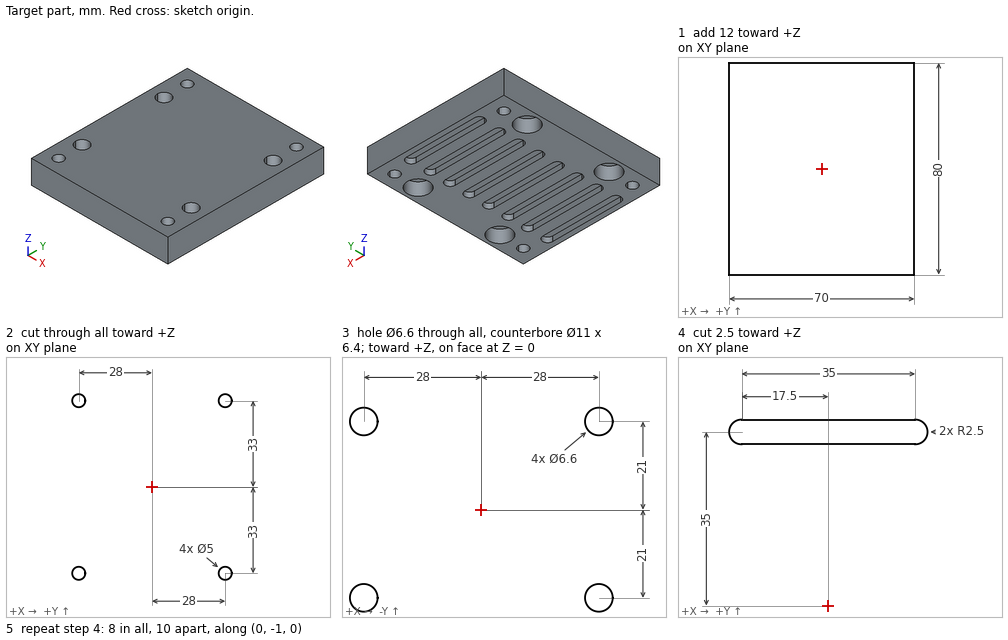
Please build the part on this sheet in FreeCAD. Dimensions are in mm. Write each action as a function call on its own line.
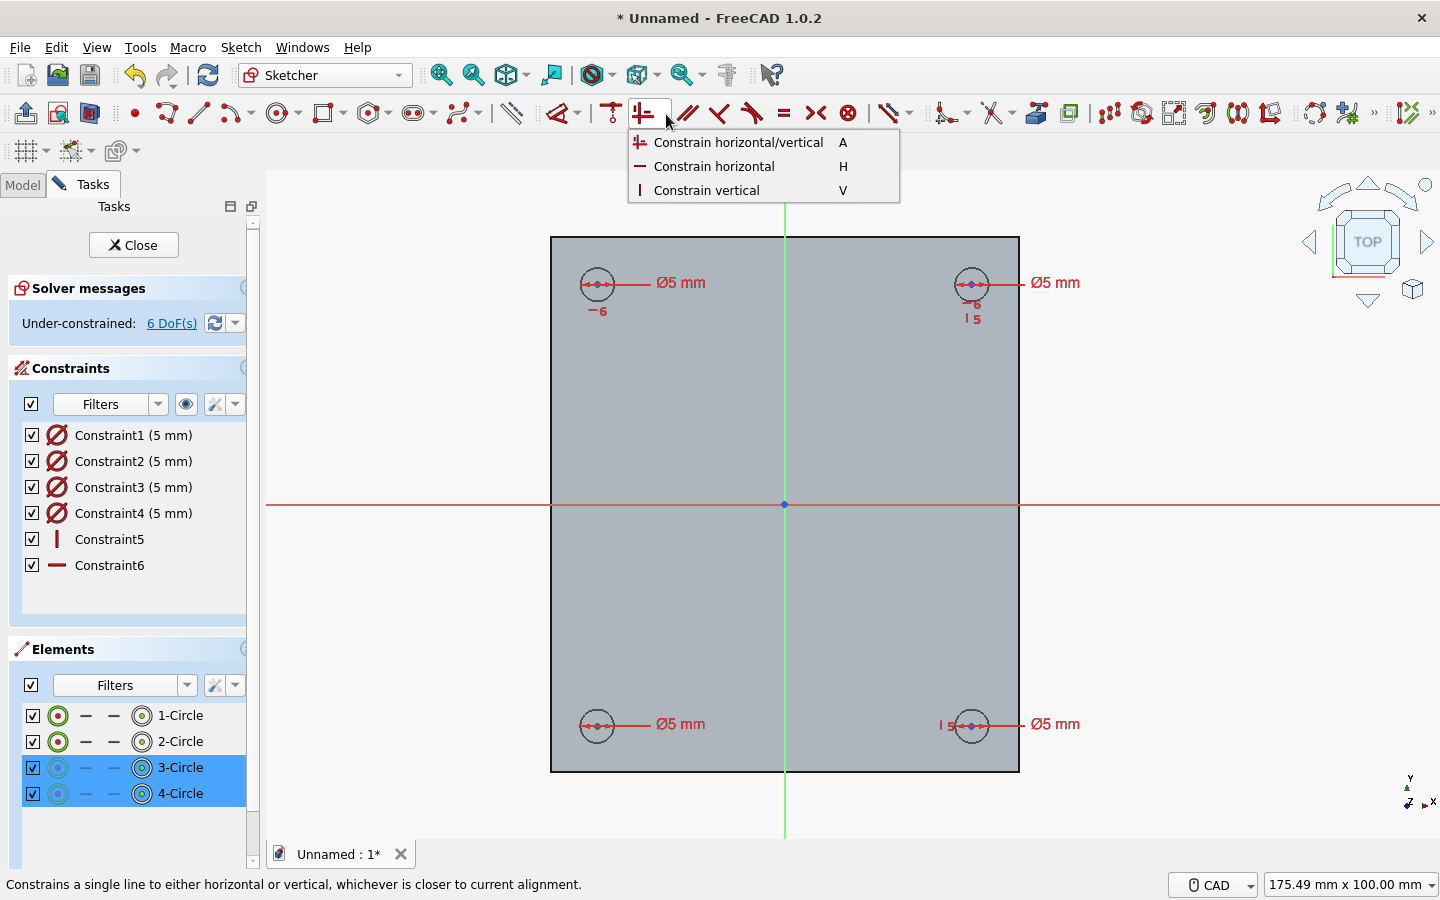
click(764, 190)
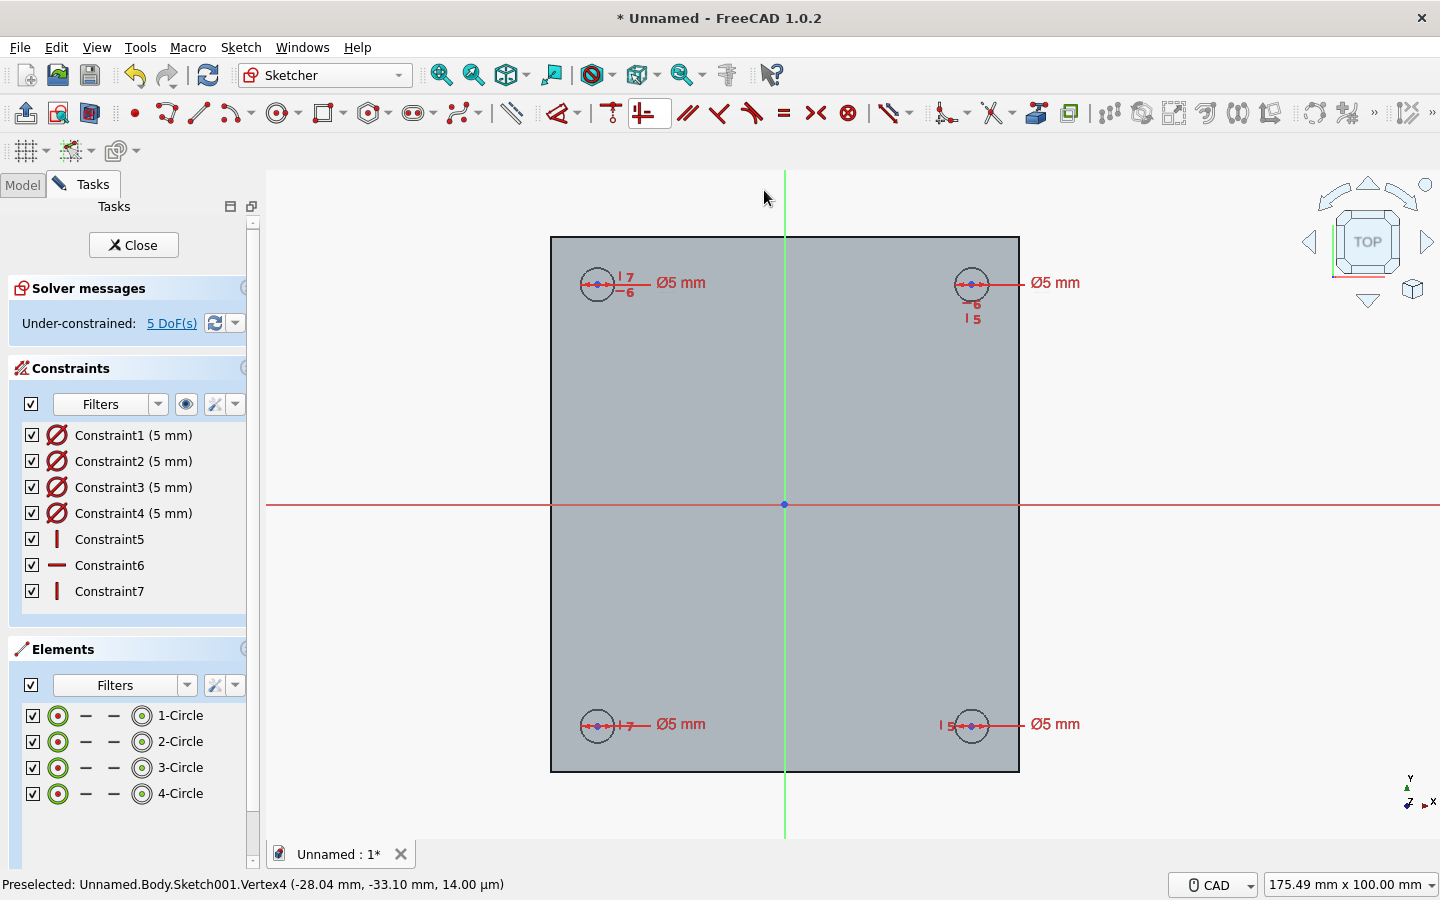
click(972, 726)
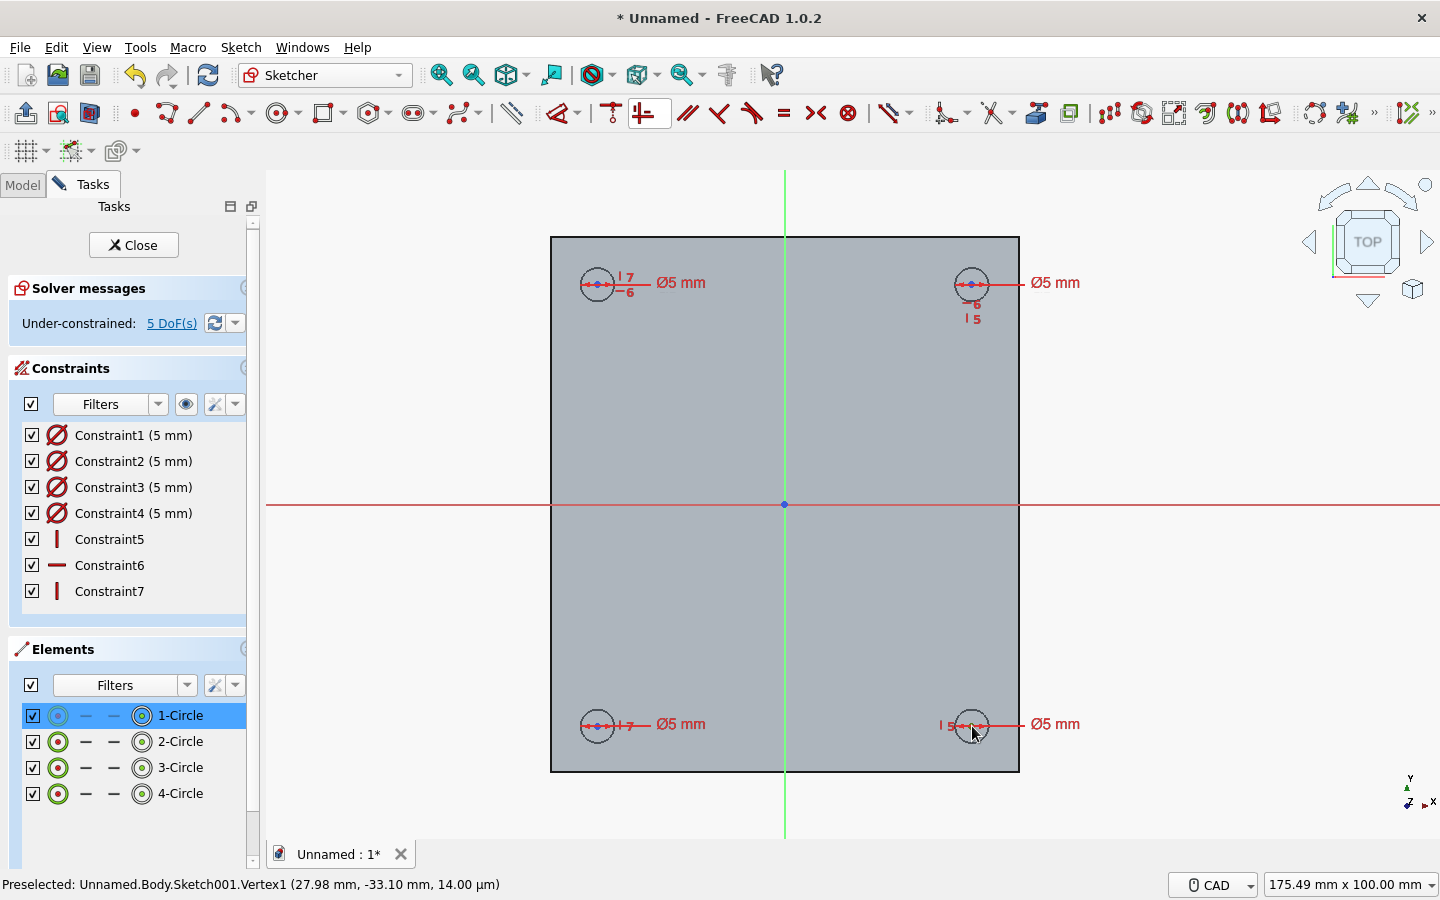
click(597, 726)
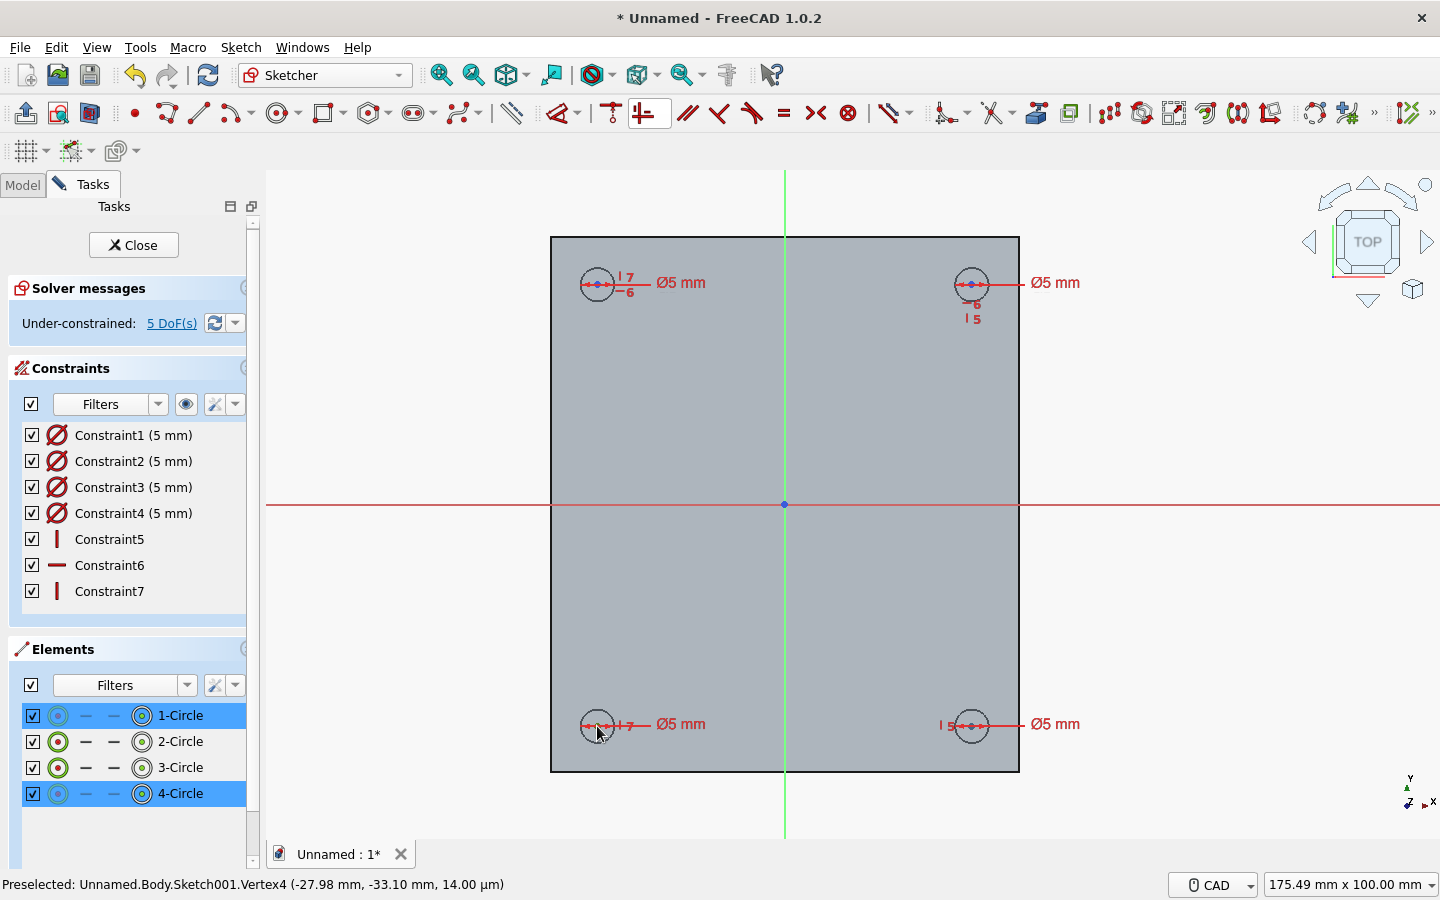
click(666, 114)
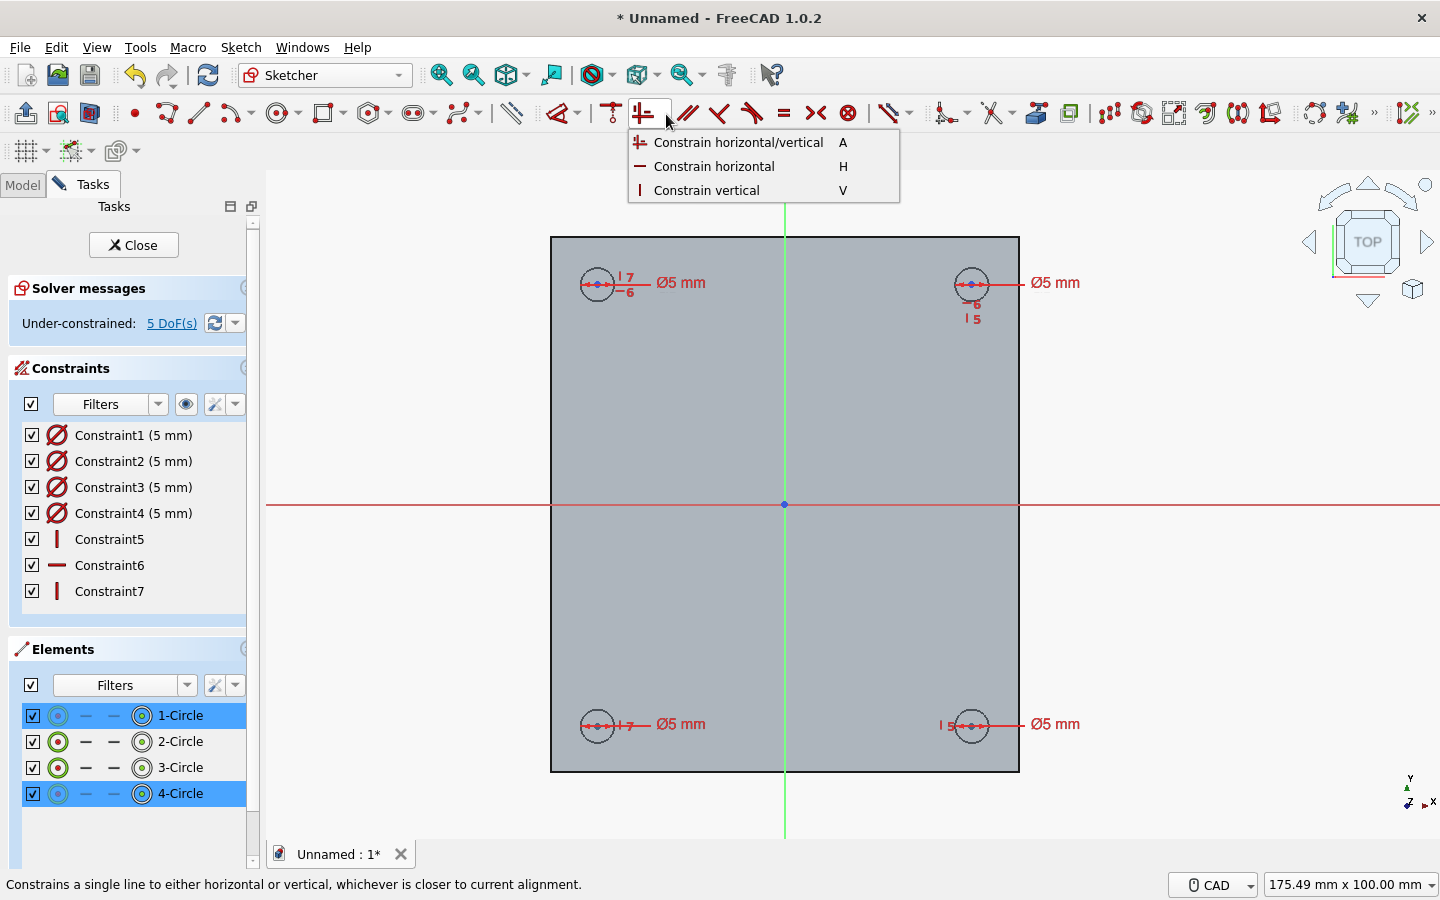
click(764, 166)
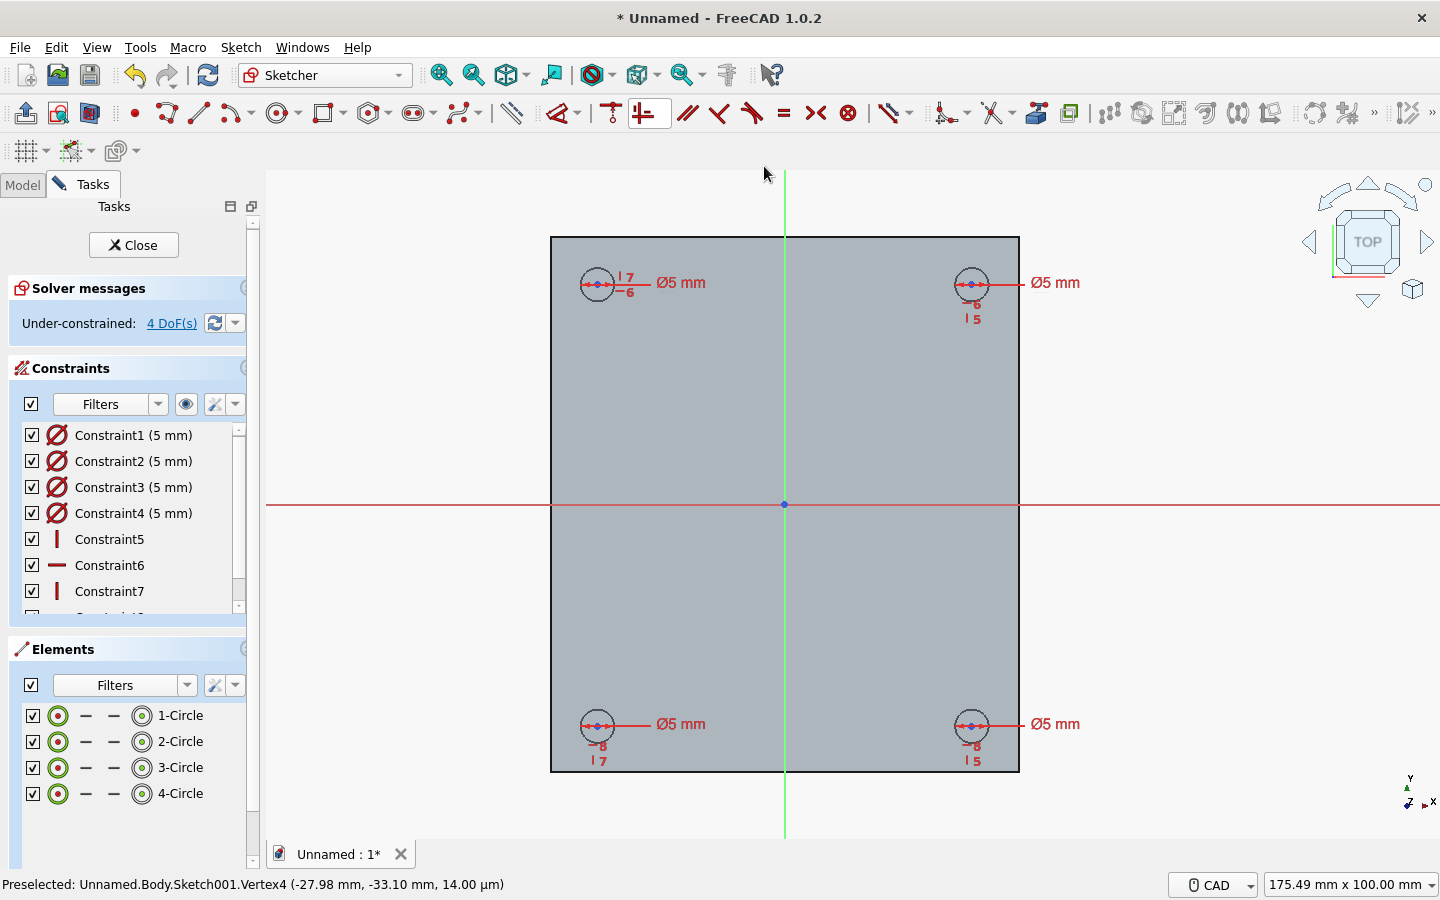
click(558, 114)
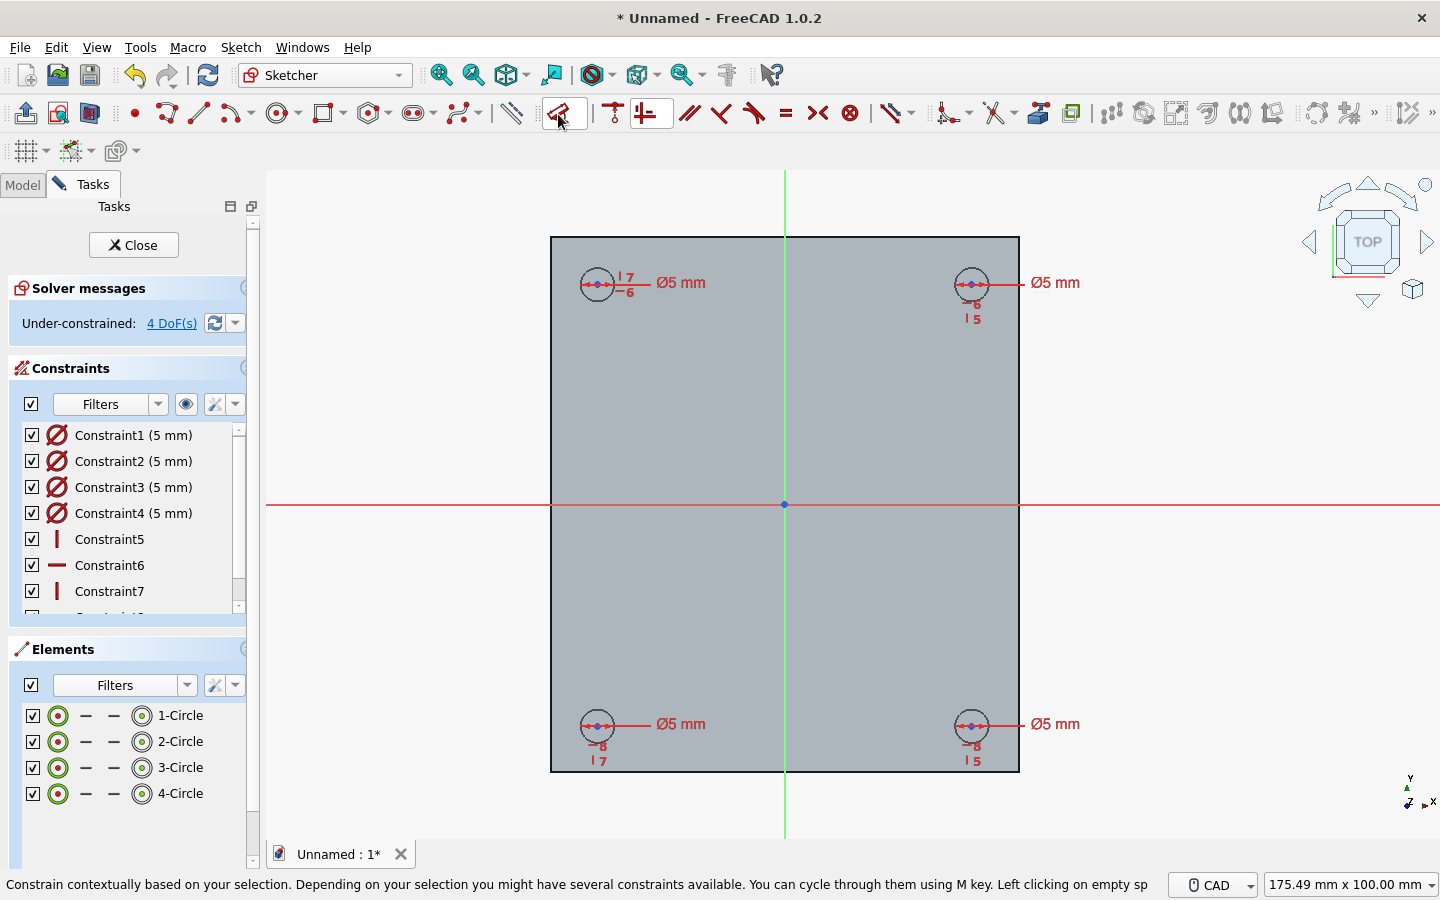
click(972, 726)
click(878, 760)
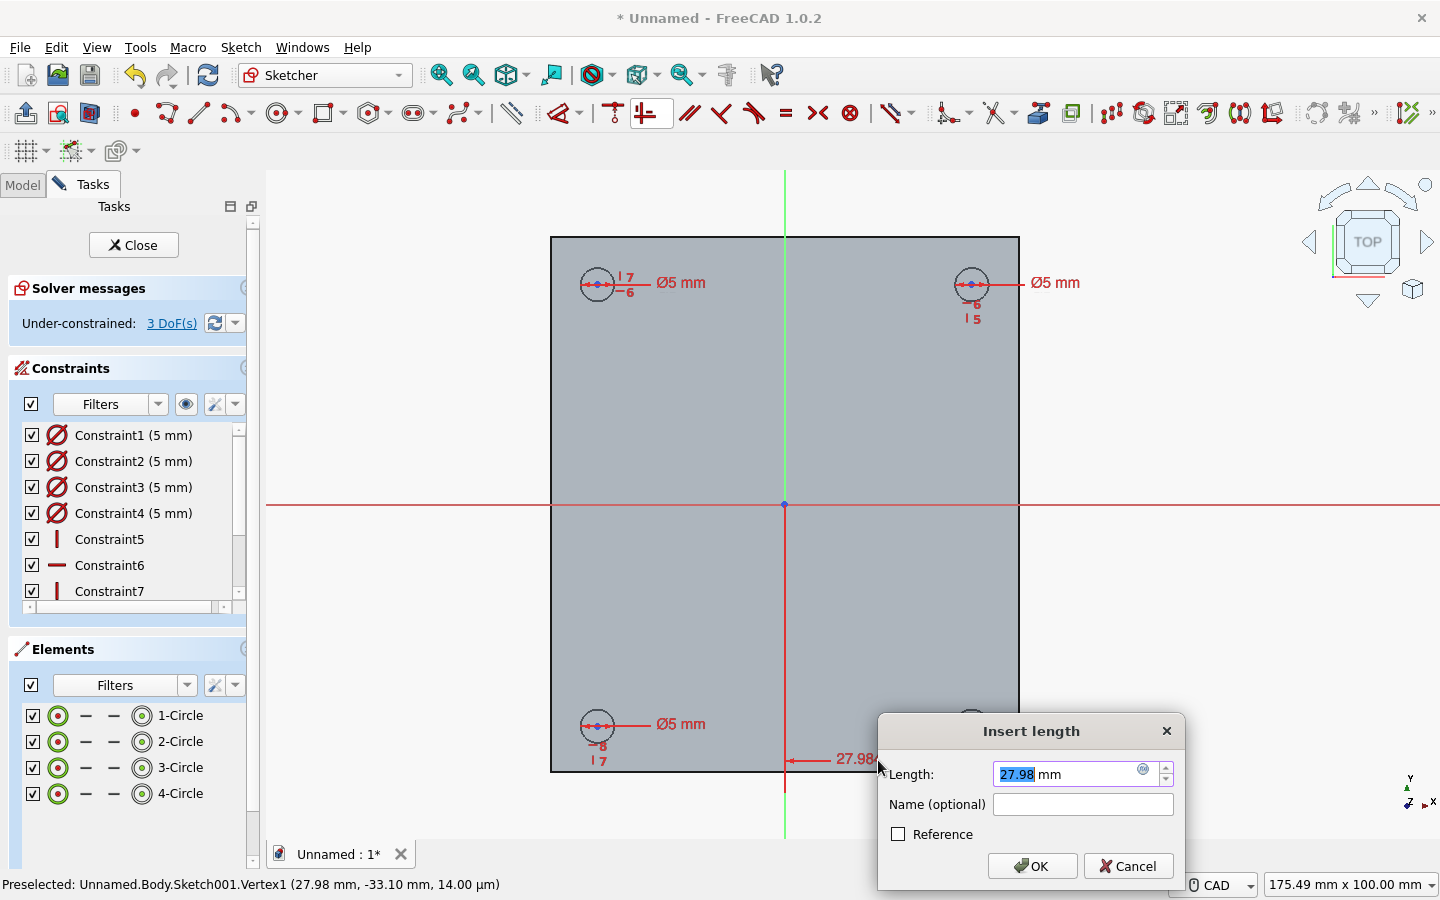
text(28)
key(Return)